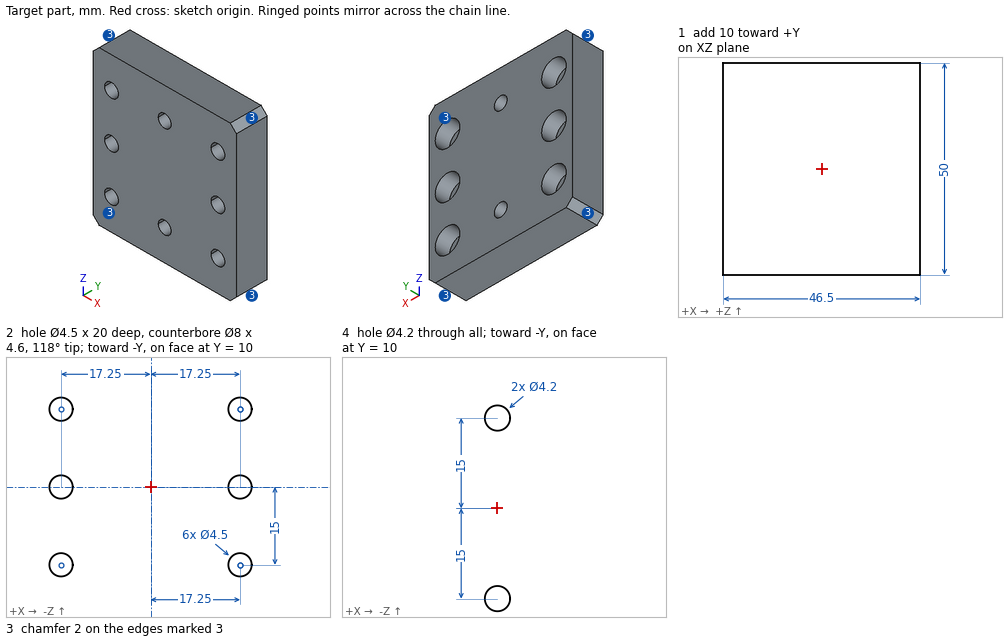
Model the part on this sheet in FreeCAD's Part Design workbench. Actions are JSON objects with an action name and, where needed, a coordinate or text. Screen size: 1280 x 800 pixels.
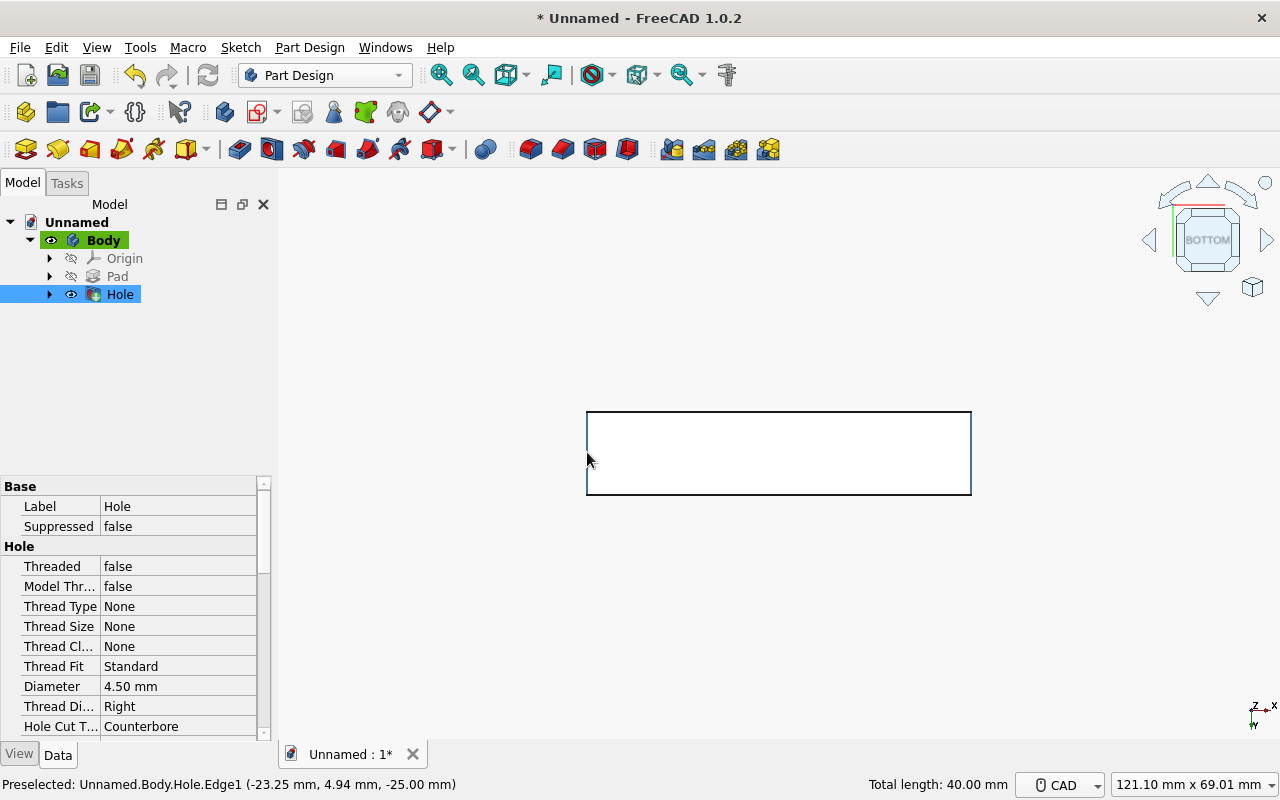
{"action": "left_click", "coordinate": [564, 150]}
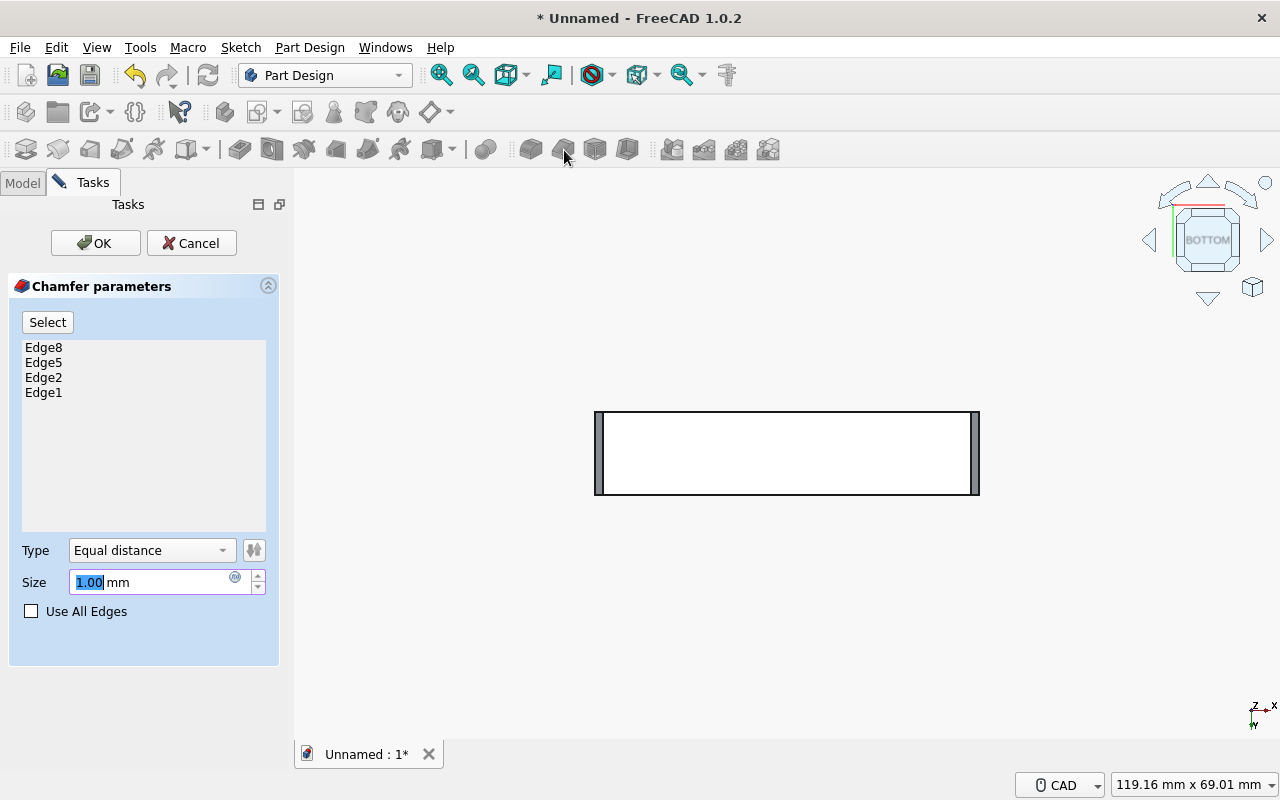
{"action": "type", "text": "2"}
{"action": "key", "text": "Tab"}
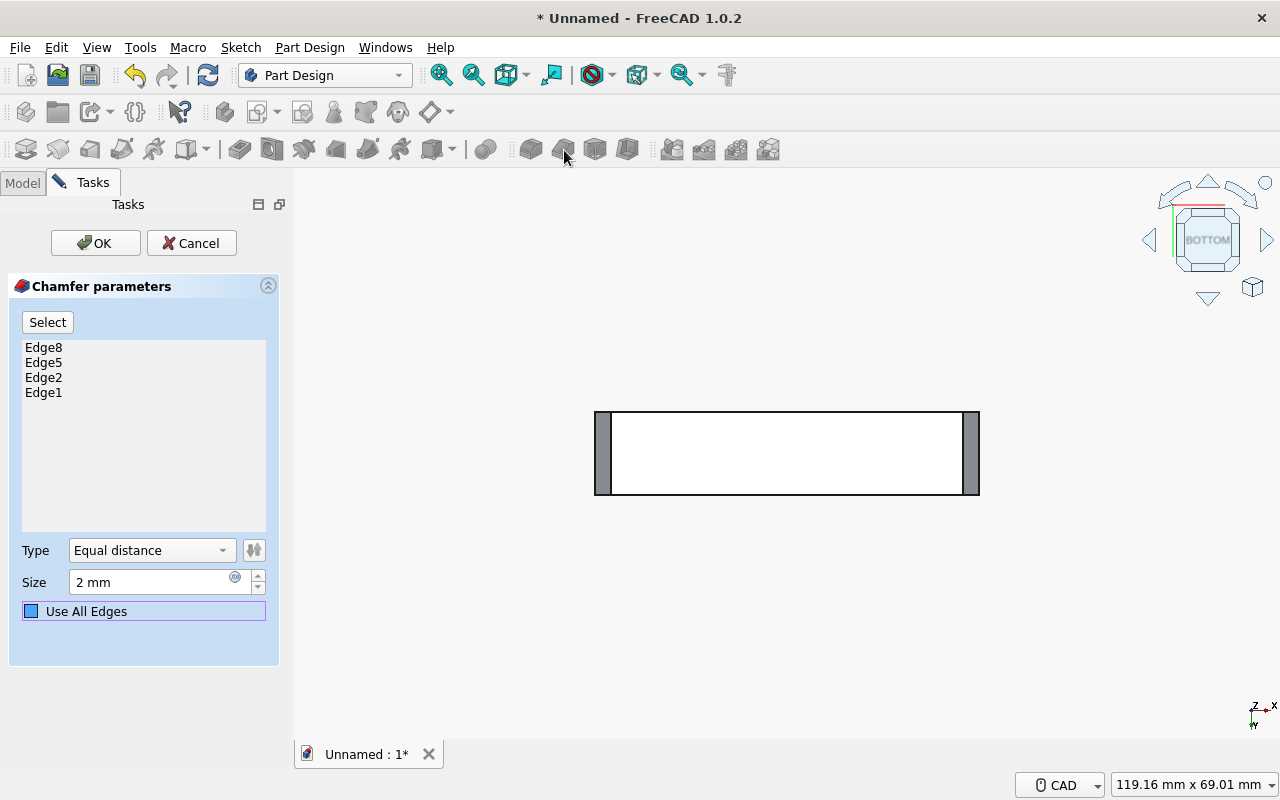
{"action": "left_click", "coordinate": [96, 243]}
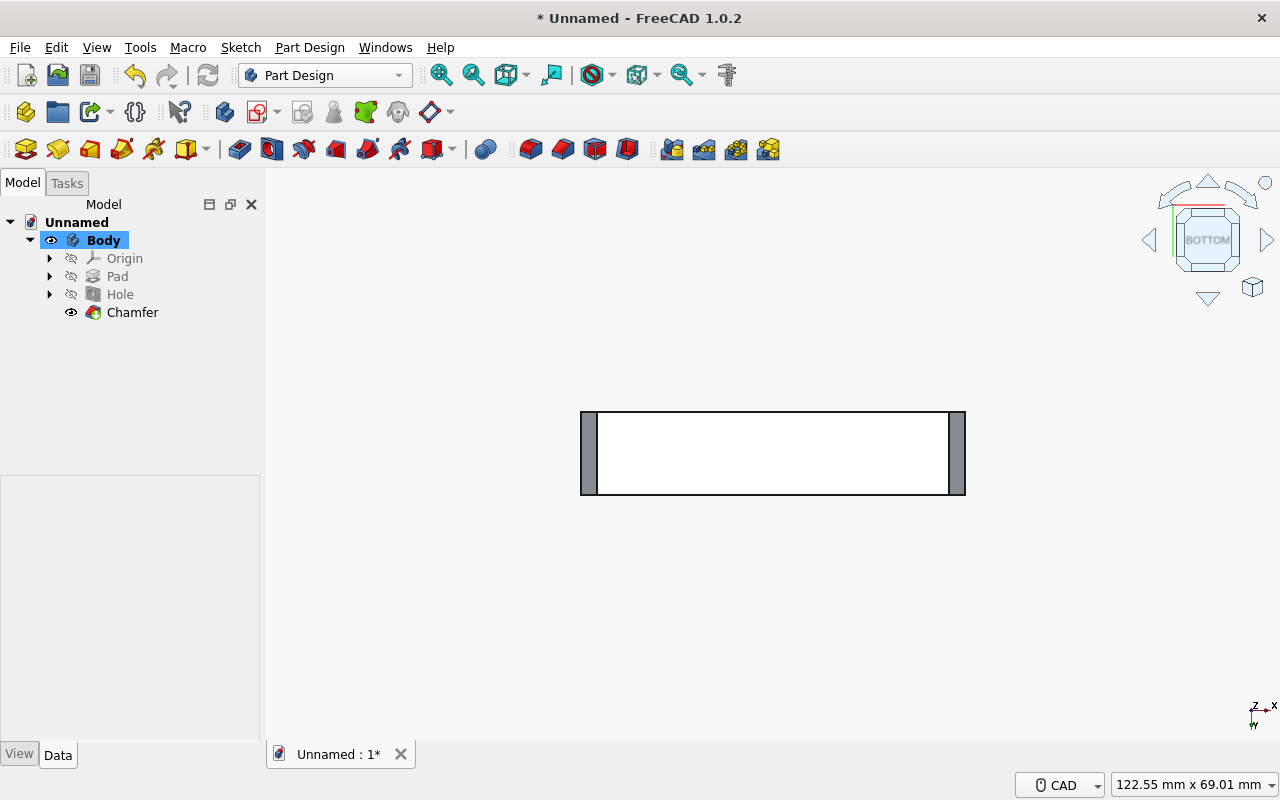
{"action": "left_click", "coordinate": [442, 76]}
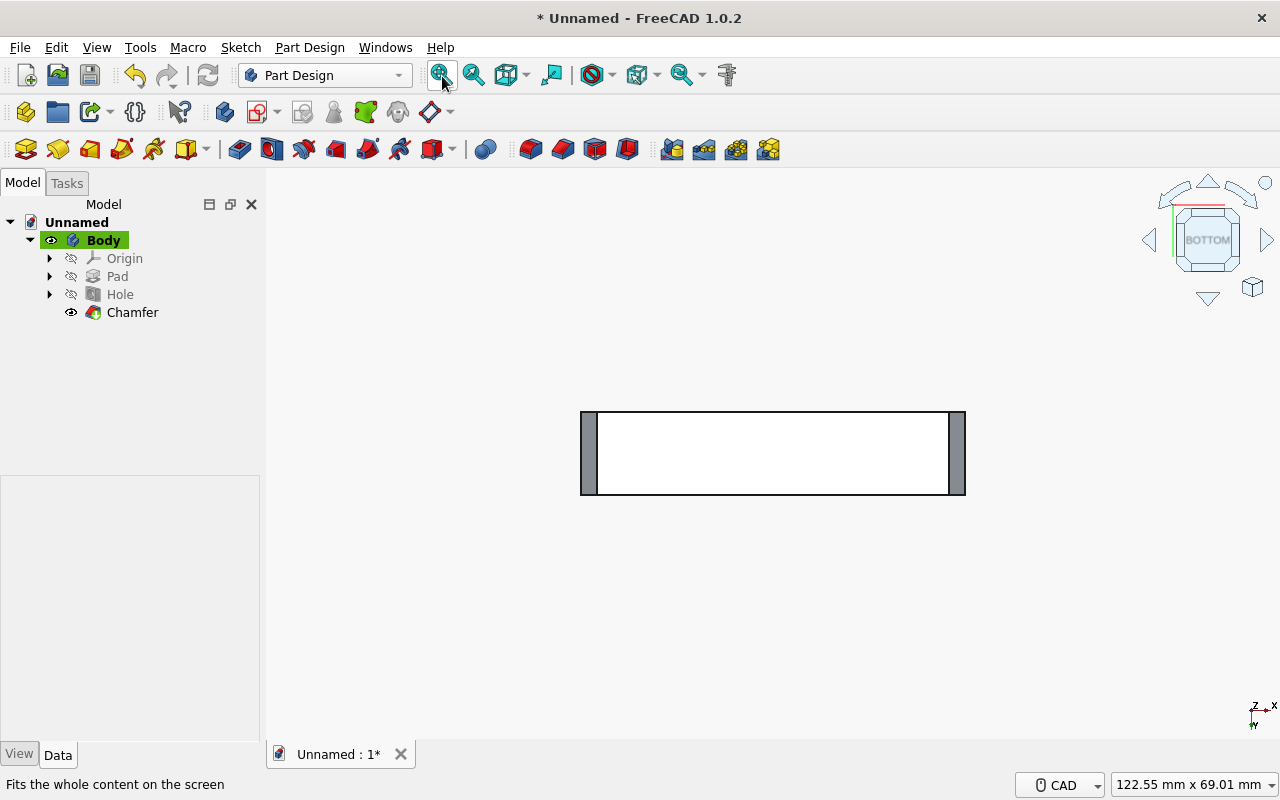
{"action": "key", "text": "4"}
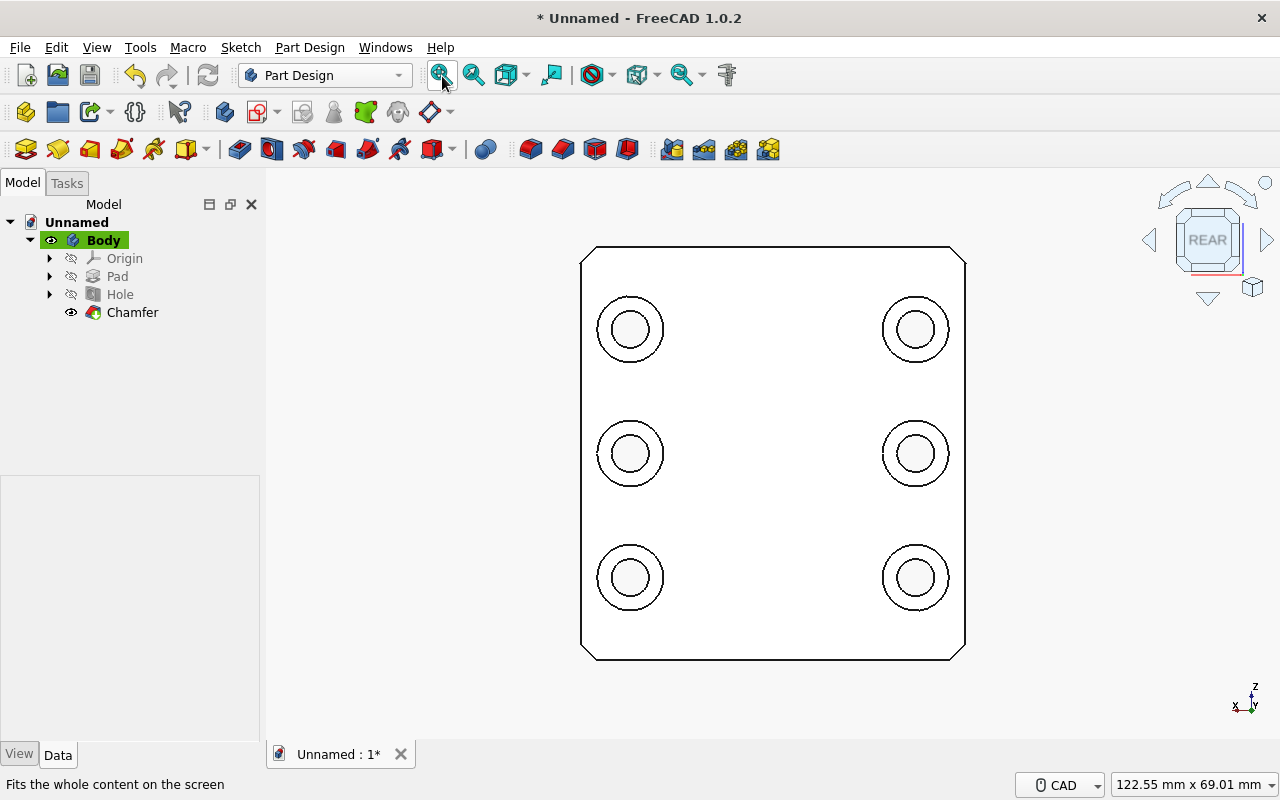
{"action": "left_click", "coordinate": [773, 393]}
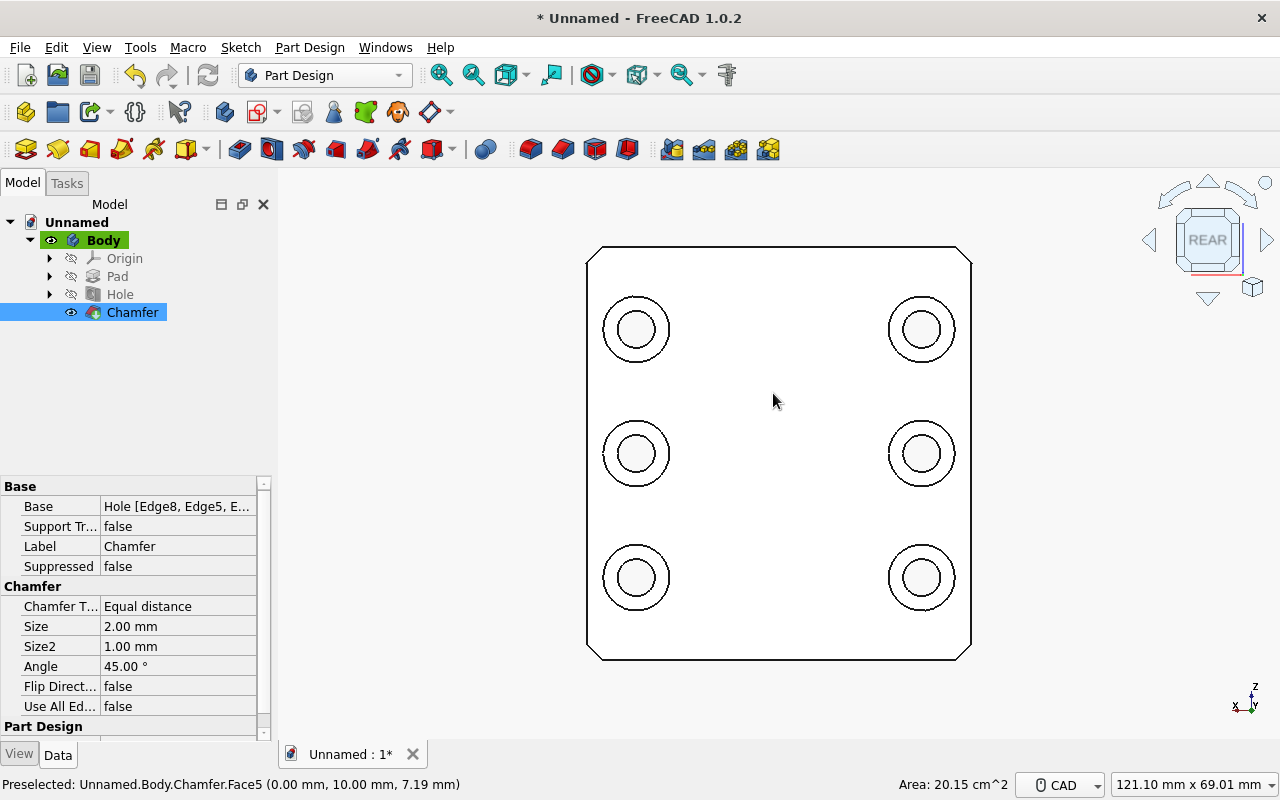
{"action": "left_click", "coordinate": [258, 112]}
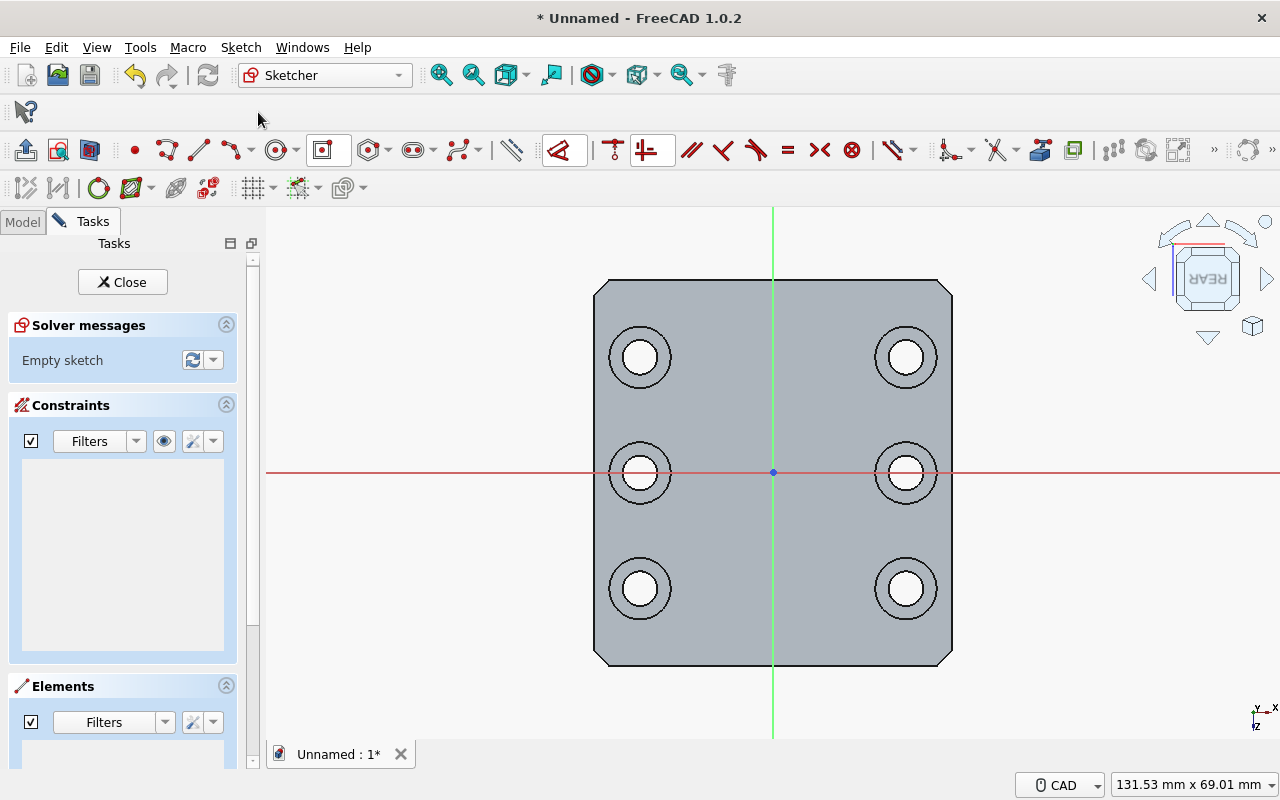
{"action": "left_click", "coordinate": [276, 150]}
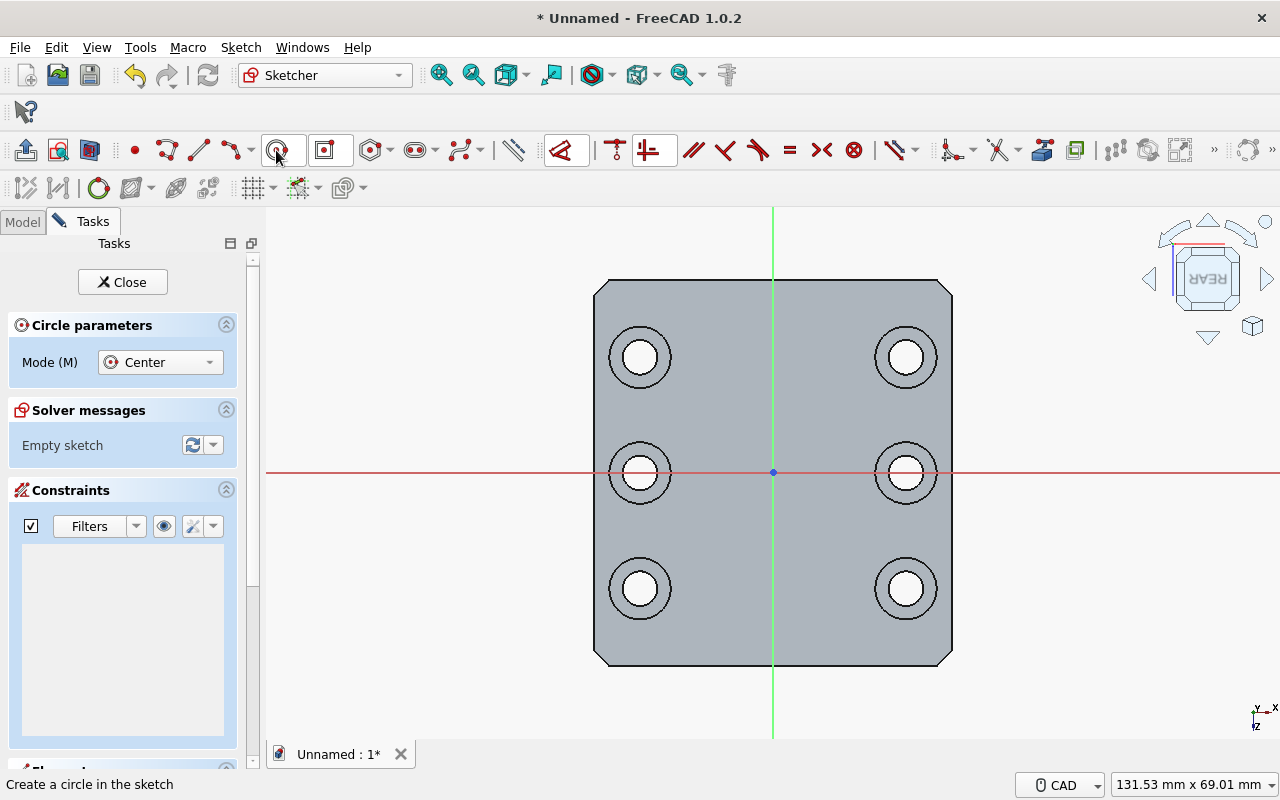
{"action": "scroll", "coordinate": [773, 357], "scroll_direction": "up", "scroll_amount": 2}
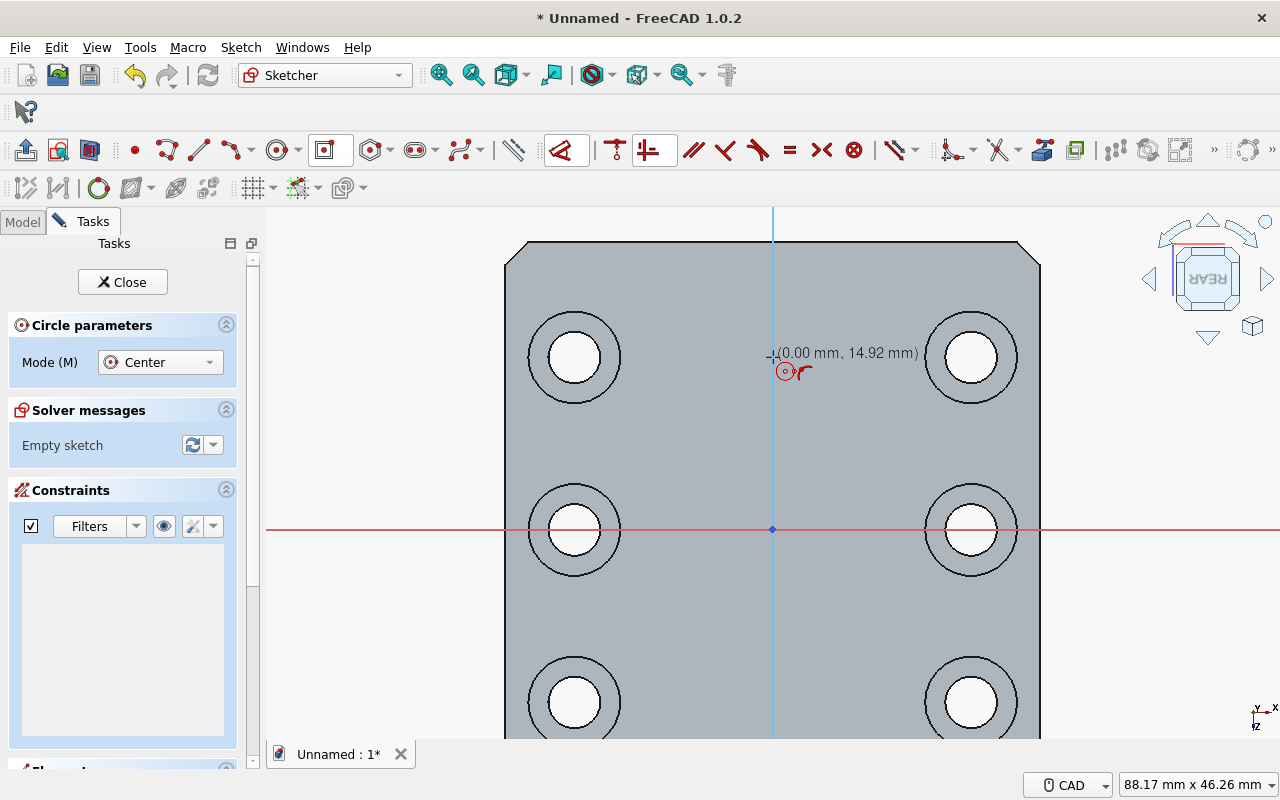
{"action": "left_click", "coordinate": [773, 357]}
{"action": "left_click", "coordinate": [790, 340]}